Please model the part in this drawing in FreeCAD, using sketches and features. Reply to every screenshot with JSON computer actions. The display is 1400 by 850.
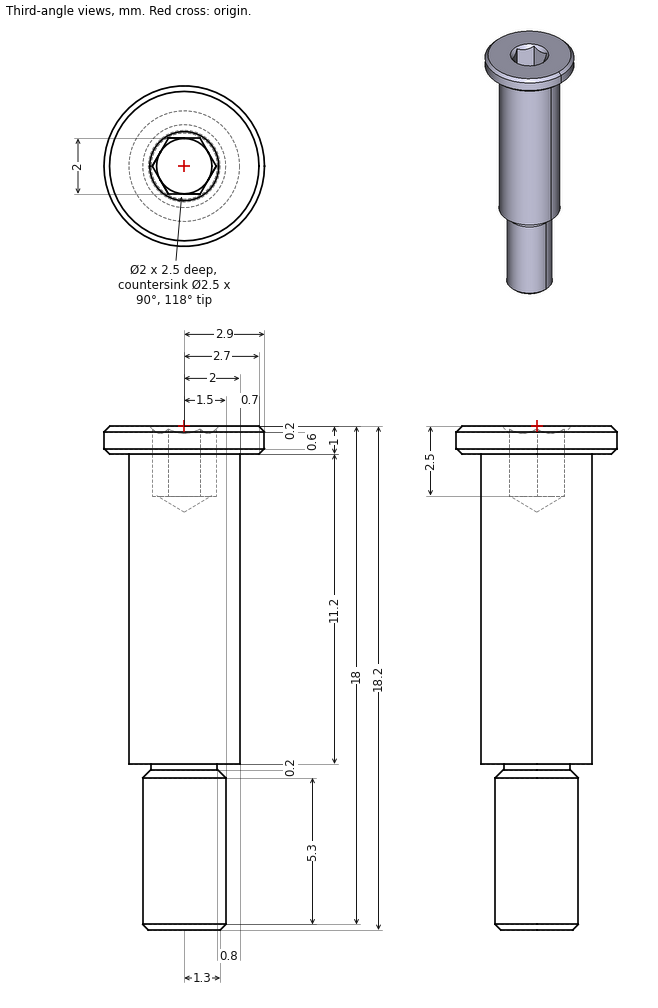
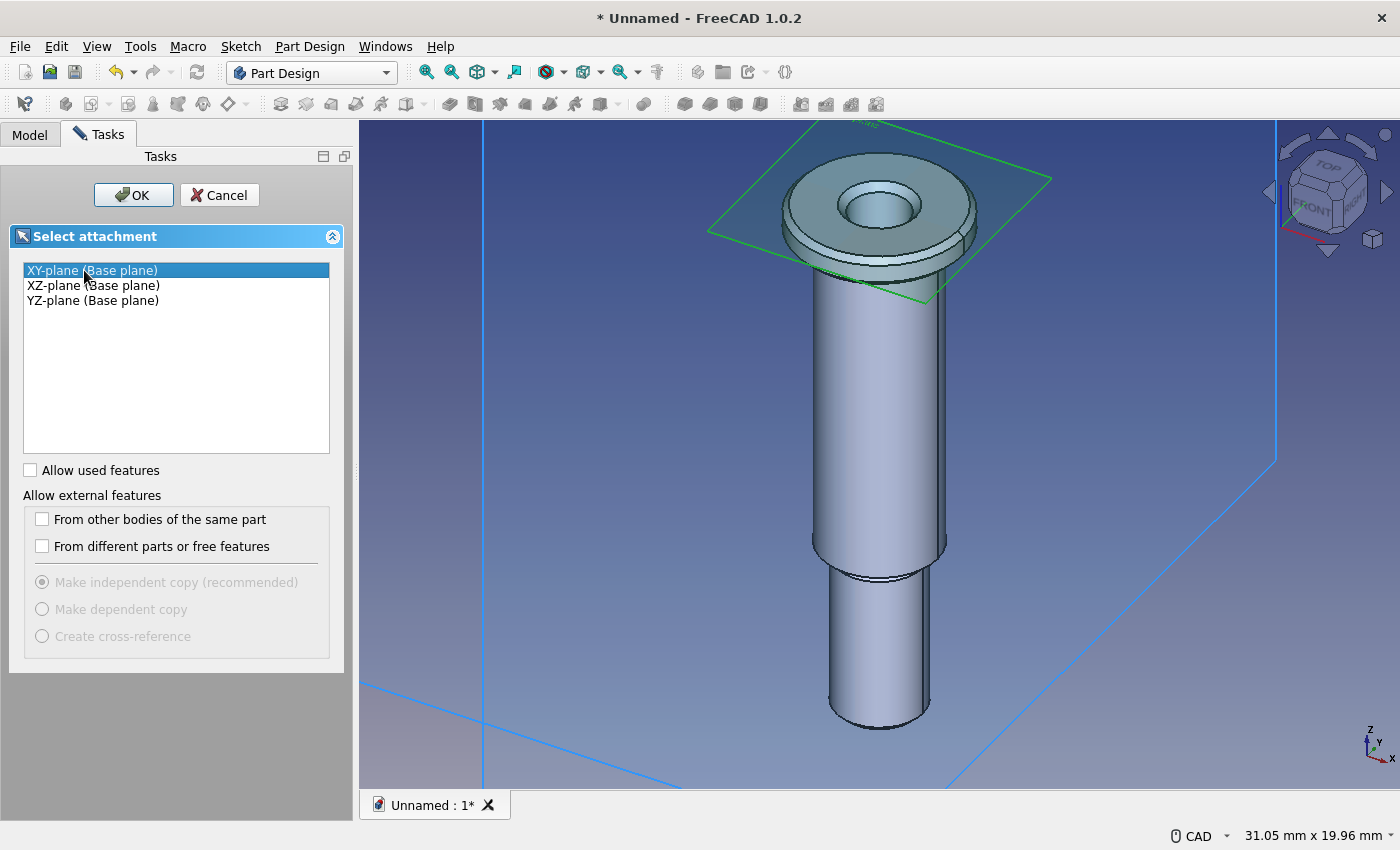
{"action": "left_click", "coordinate": [134, 195]}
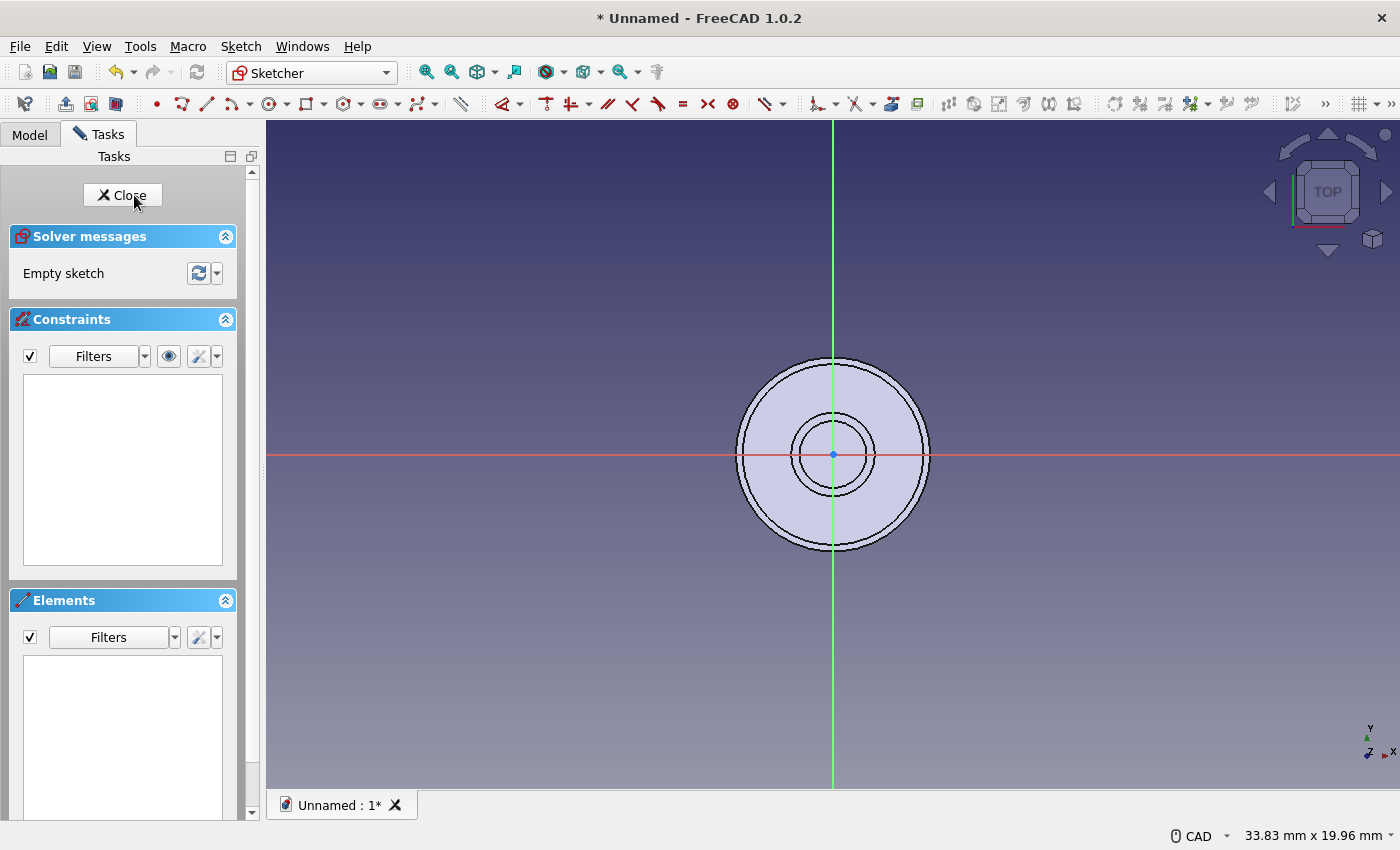
{"action": "scroll", "coordinate": [847, 455], "scroll_direction": "up", "scroll_amount": 9}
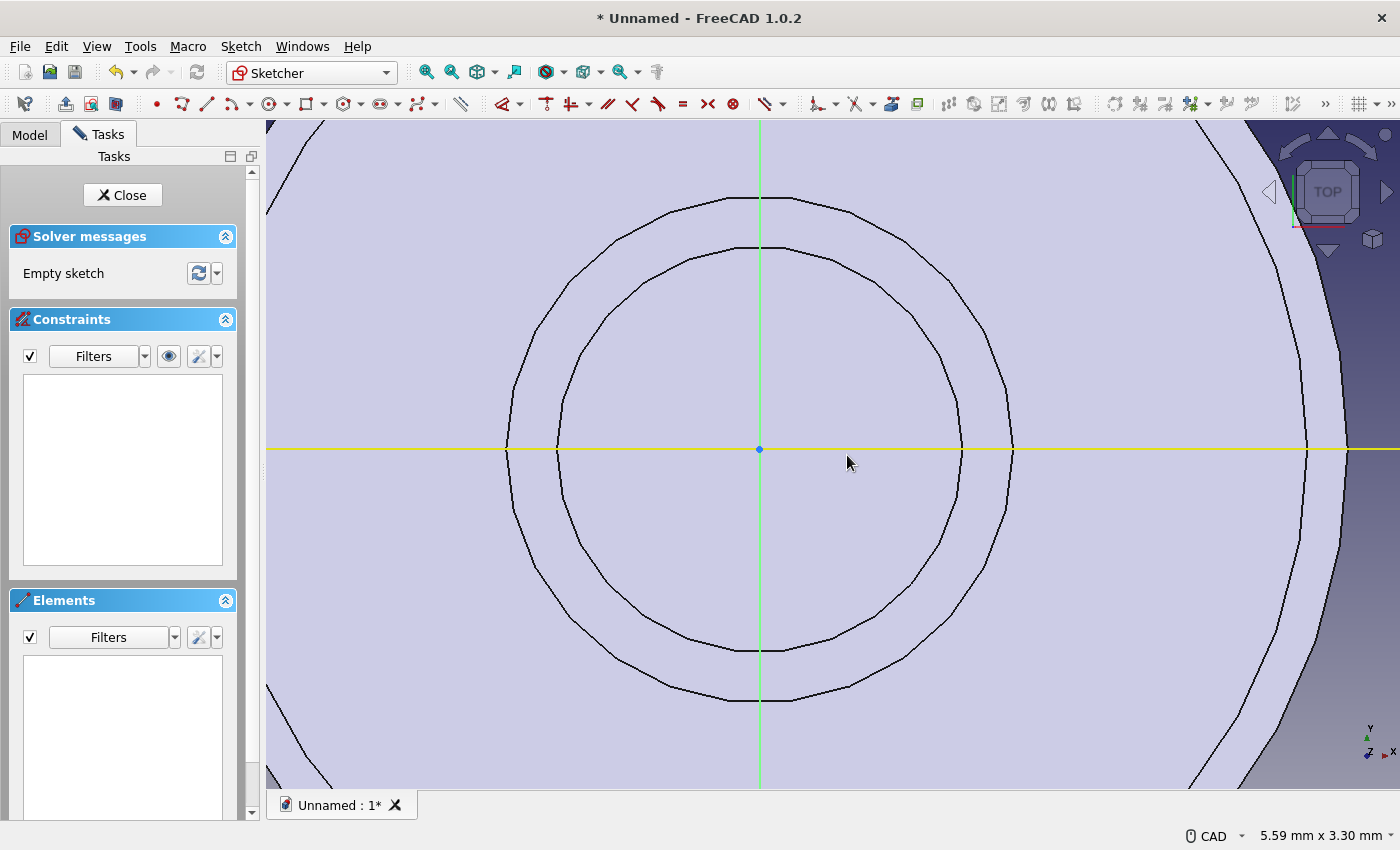
{"action": "left_click", "coordinate": [342, 104]}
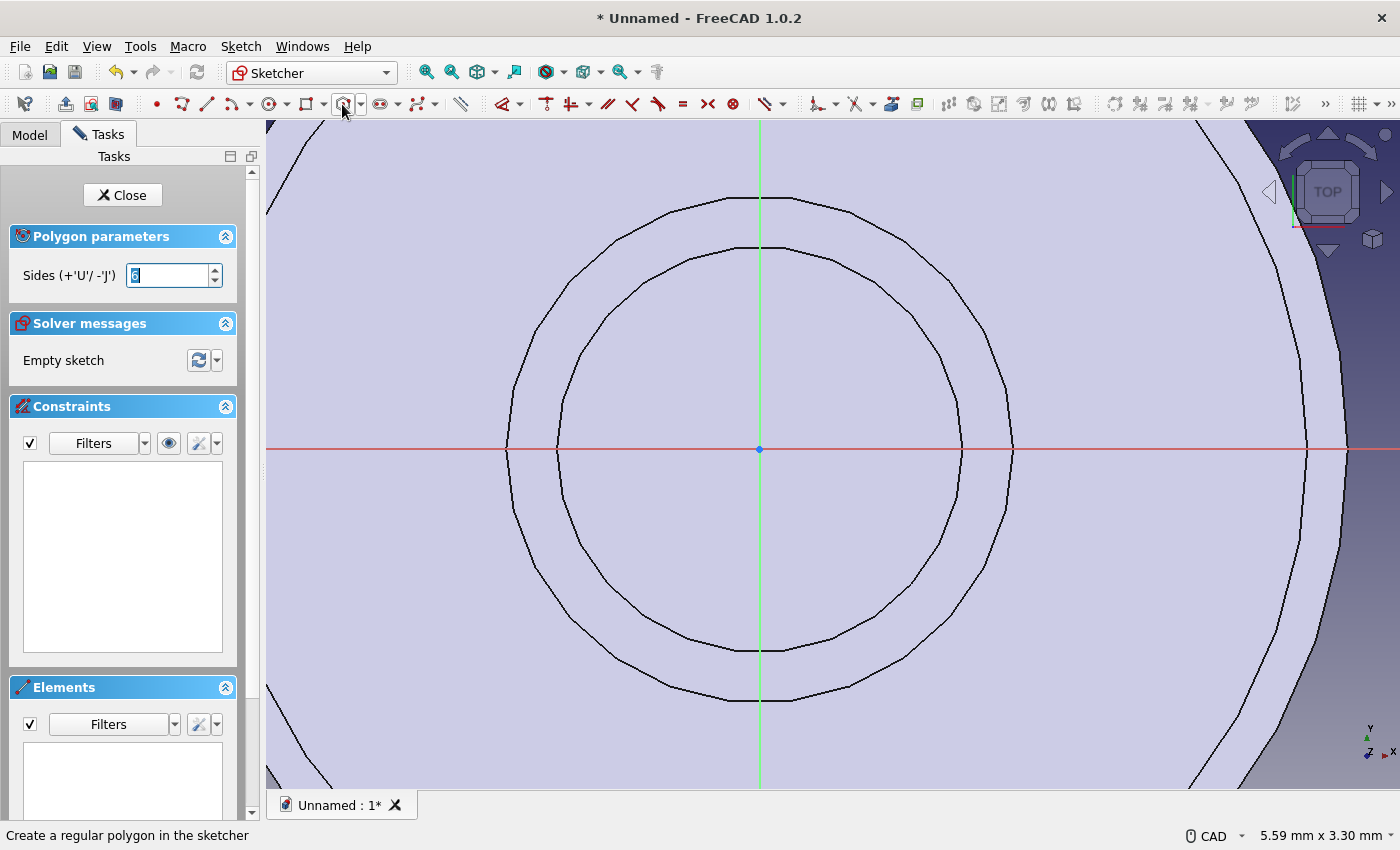
{"action": "left_click", "coordinate": [760, 449]}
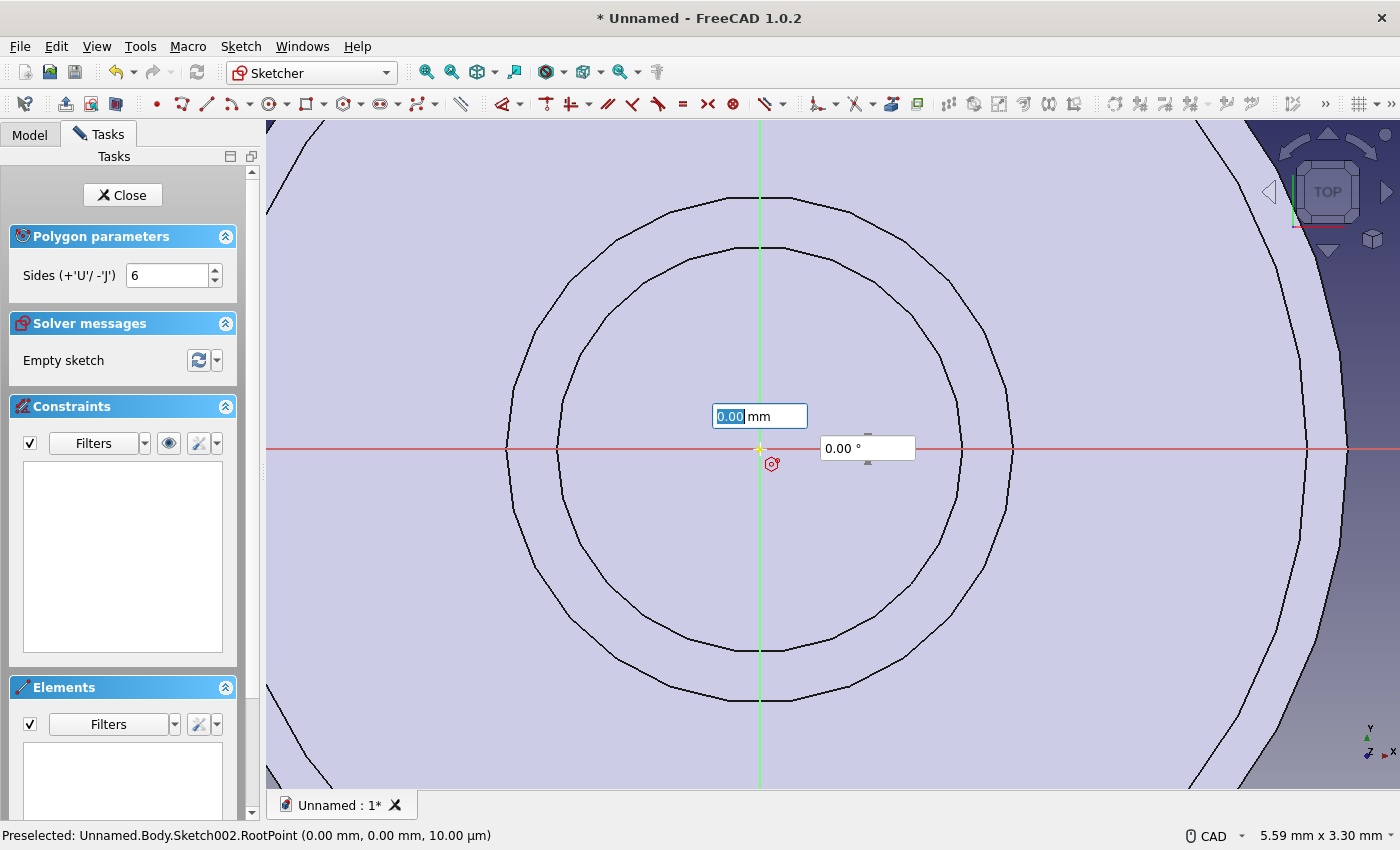
{"action": "left_click", "coordinate": [994, 449]}
{"action": "right_click", "coordinate": [994, 449]}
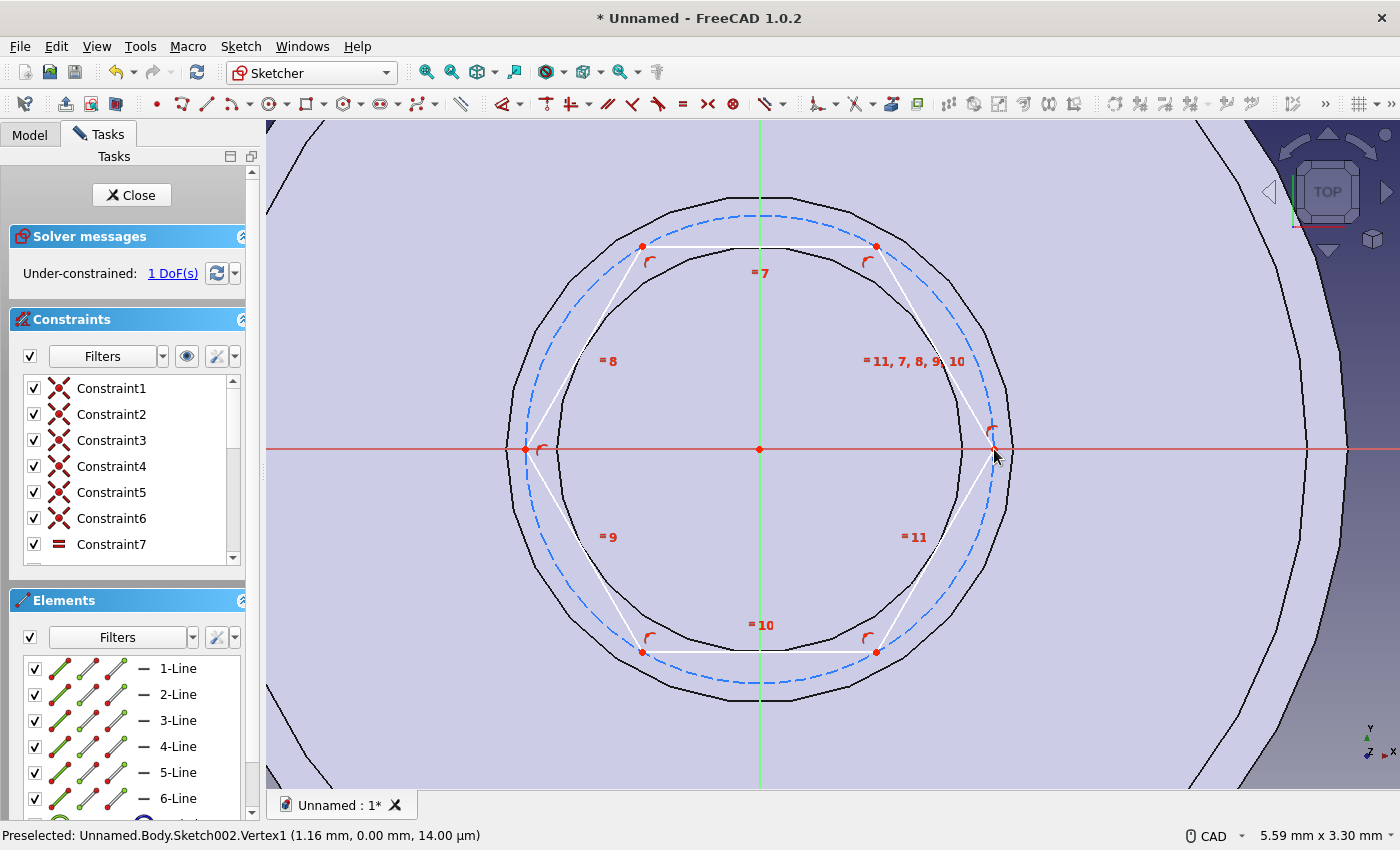
{"action": "left_click", "coordinate": [502, 104]}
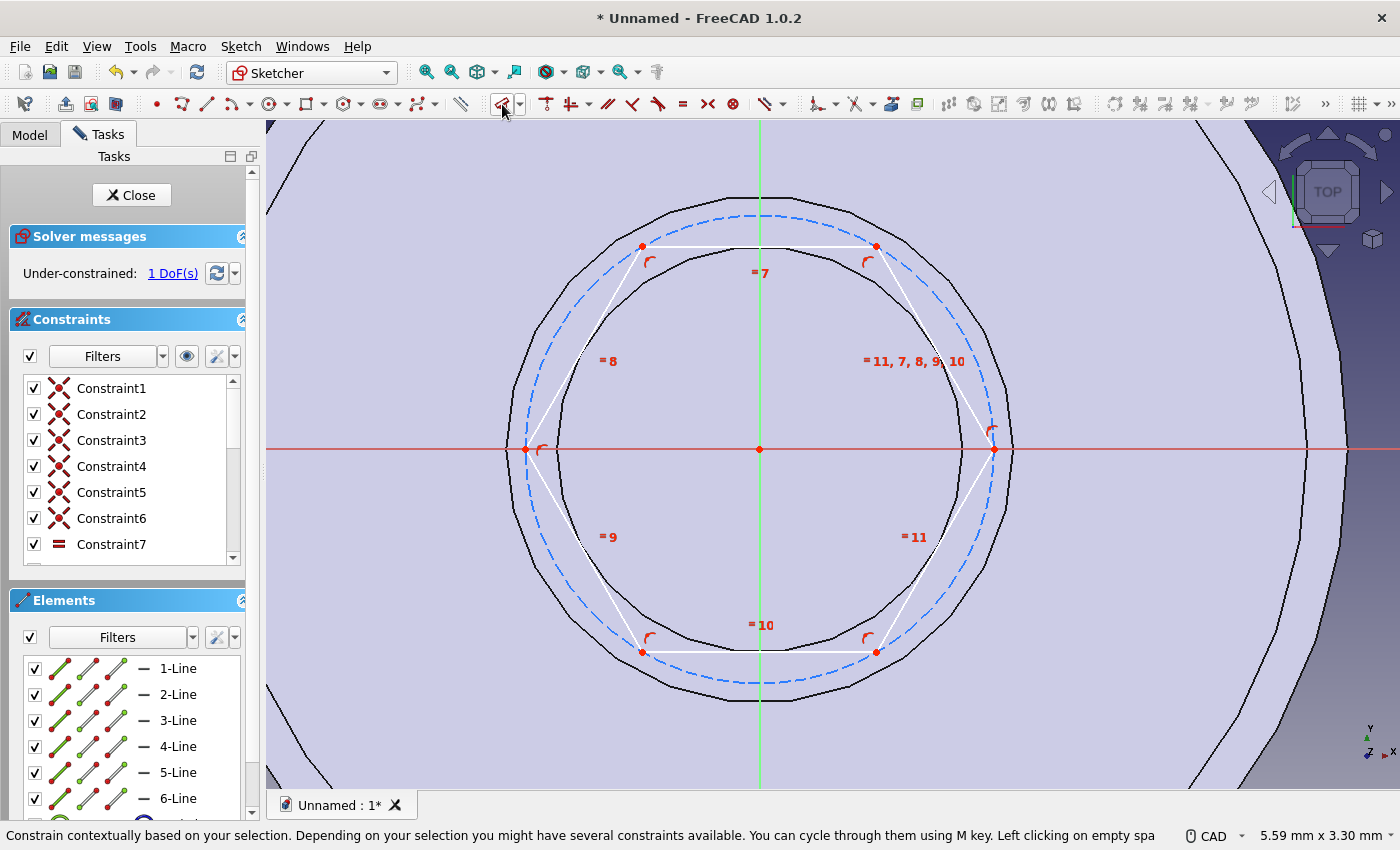
{"action": "left_click", "coordinate": [643, 652]}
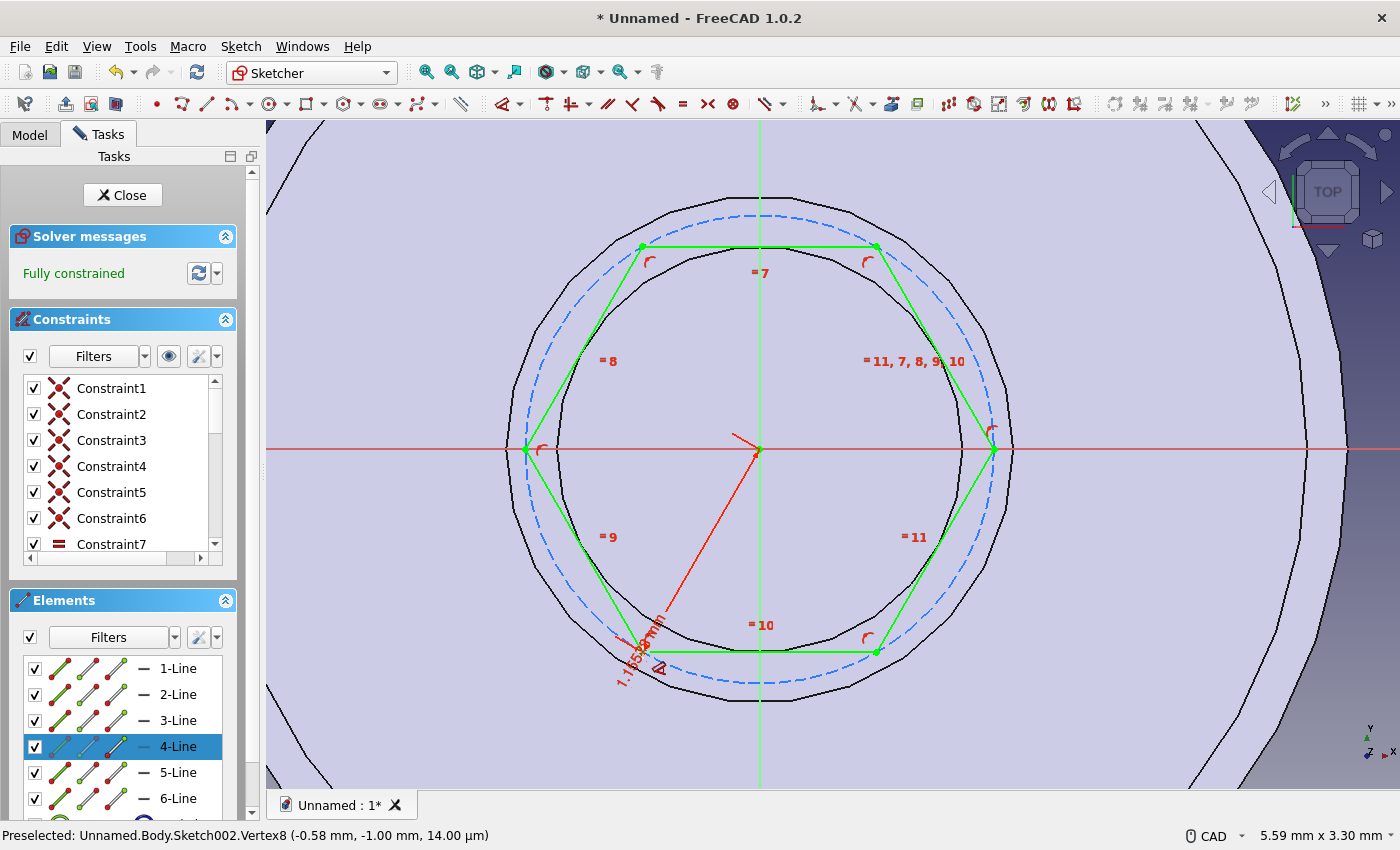
{"action": "left_click", "coordinate": [877, 247]}
{"action": "left_click", "coordinate": [911, 356]}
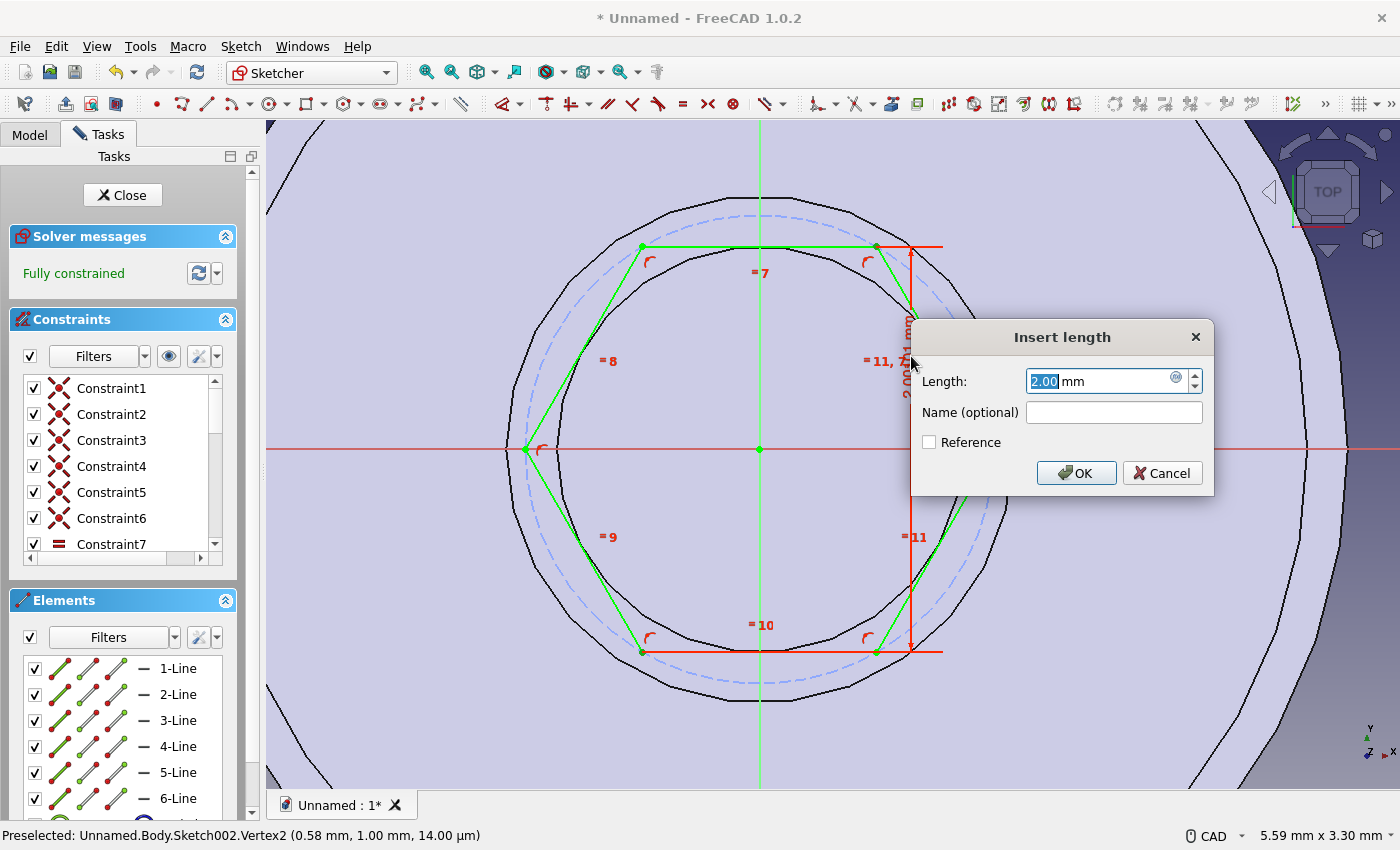
{"action": "type", "text": "2"}
{"action": "key", "text": "Return"}
{"action": "key", "text": "Escape"}